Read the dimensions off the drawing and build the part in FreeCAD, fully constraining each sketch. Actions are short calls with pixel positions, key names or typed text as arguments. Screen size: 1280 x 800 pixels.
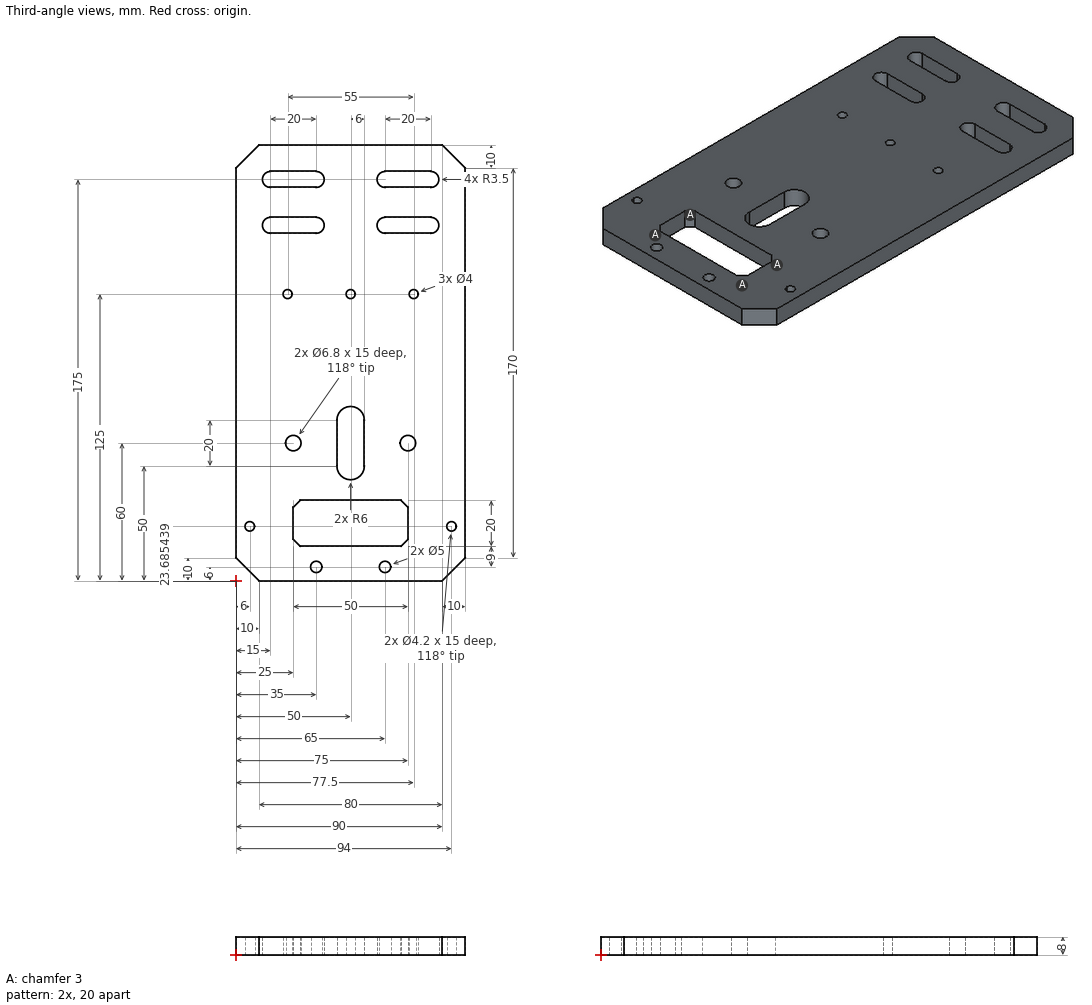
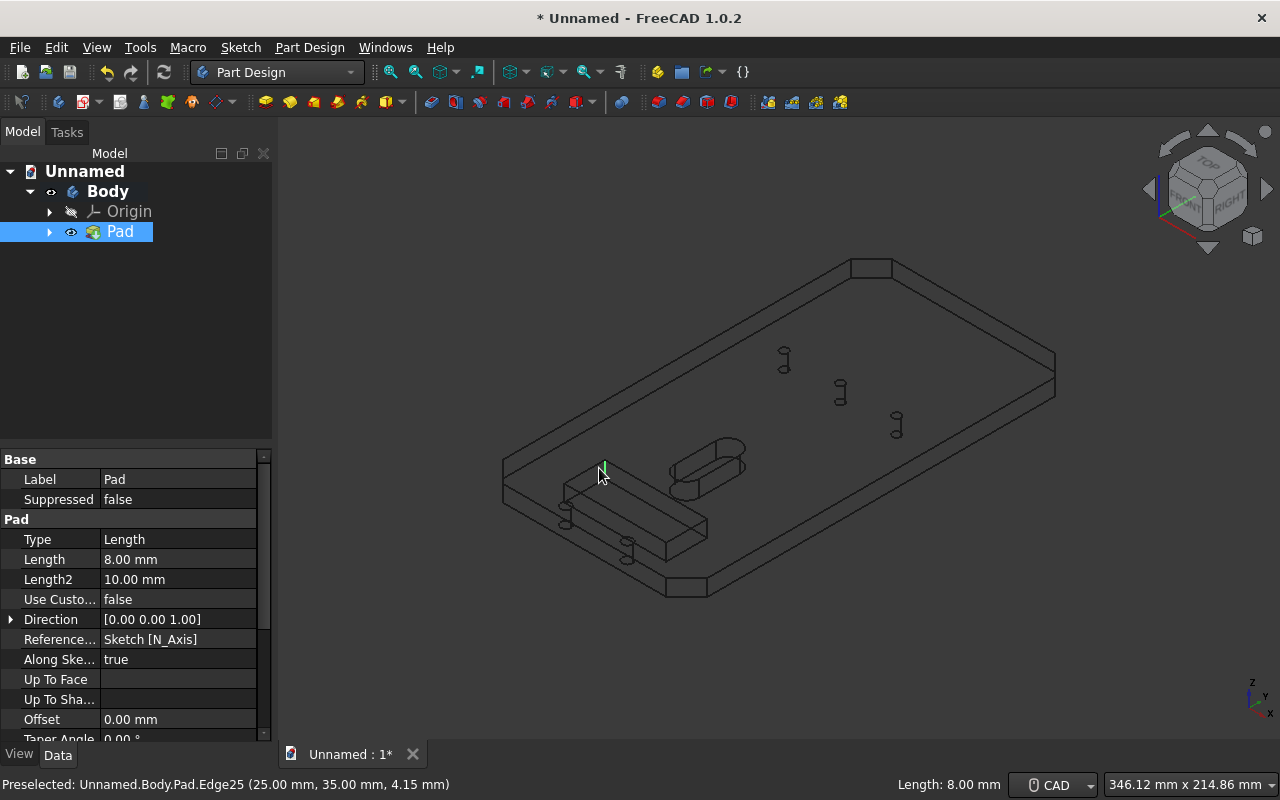
click(564, 492, ctrl)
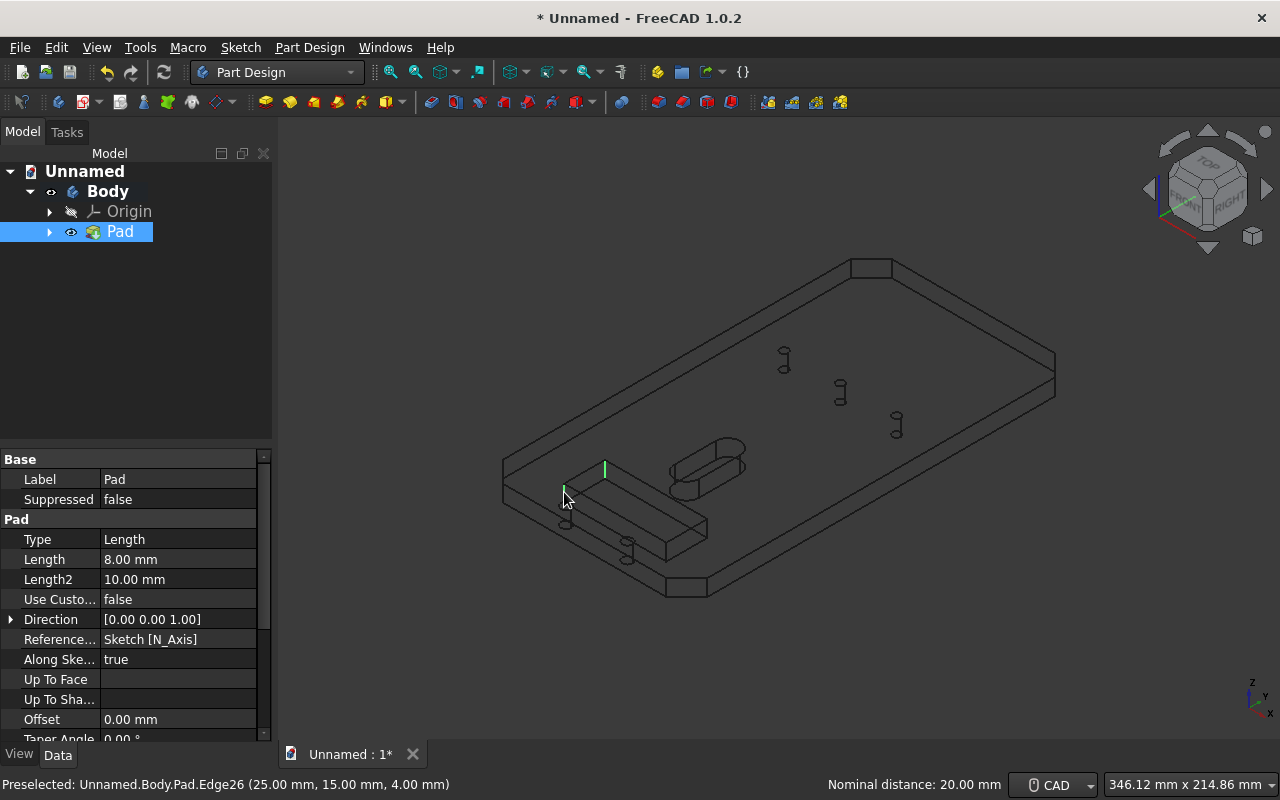
click(666, 551, ctrl)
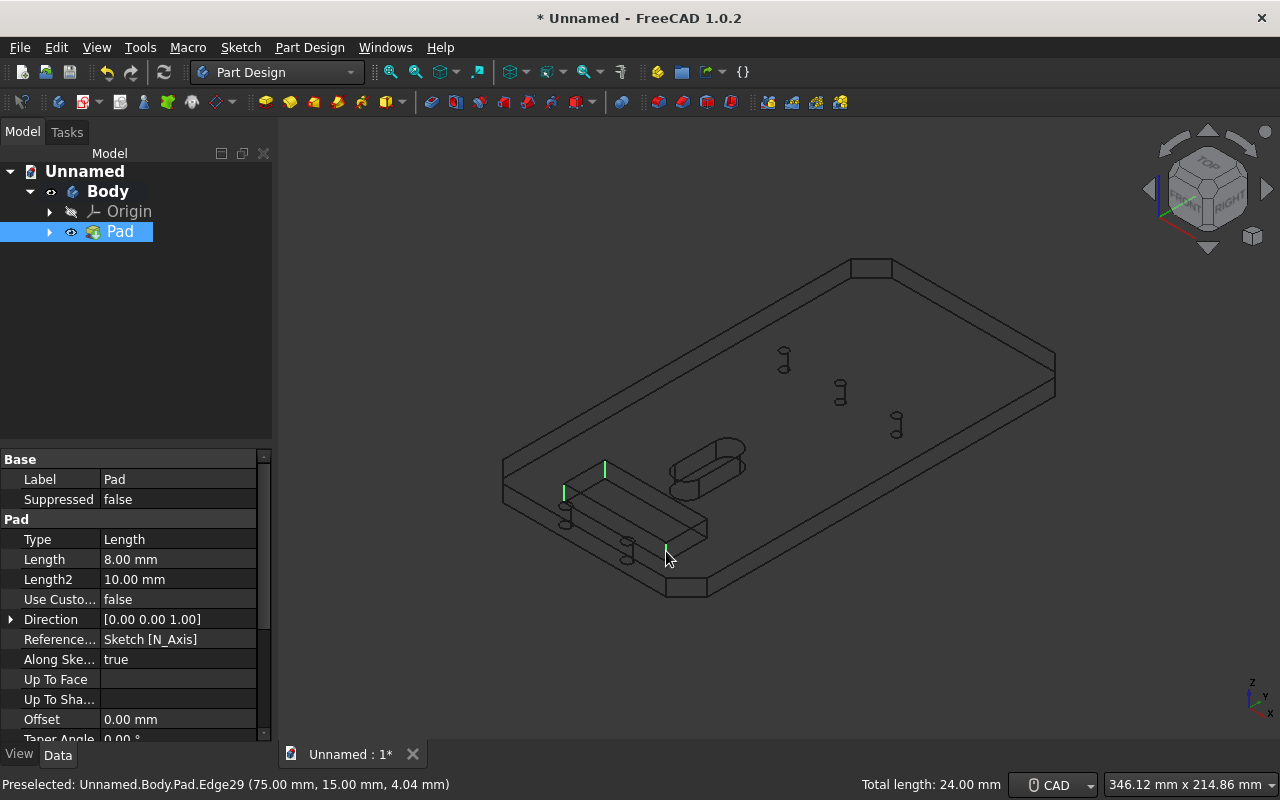
click(707, 527, ctrl)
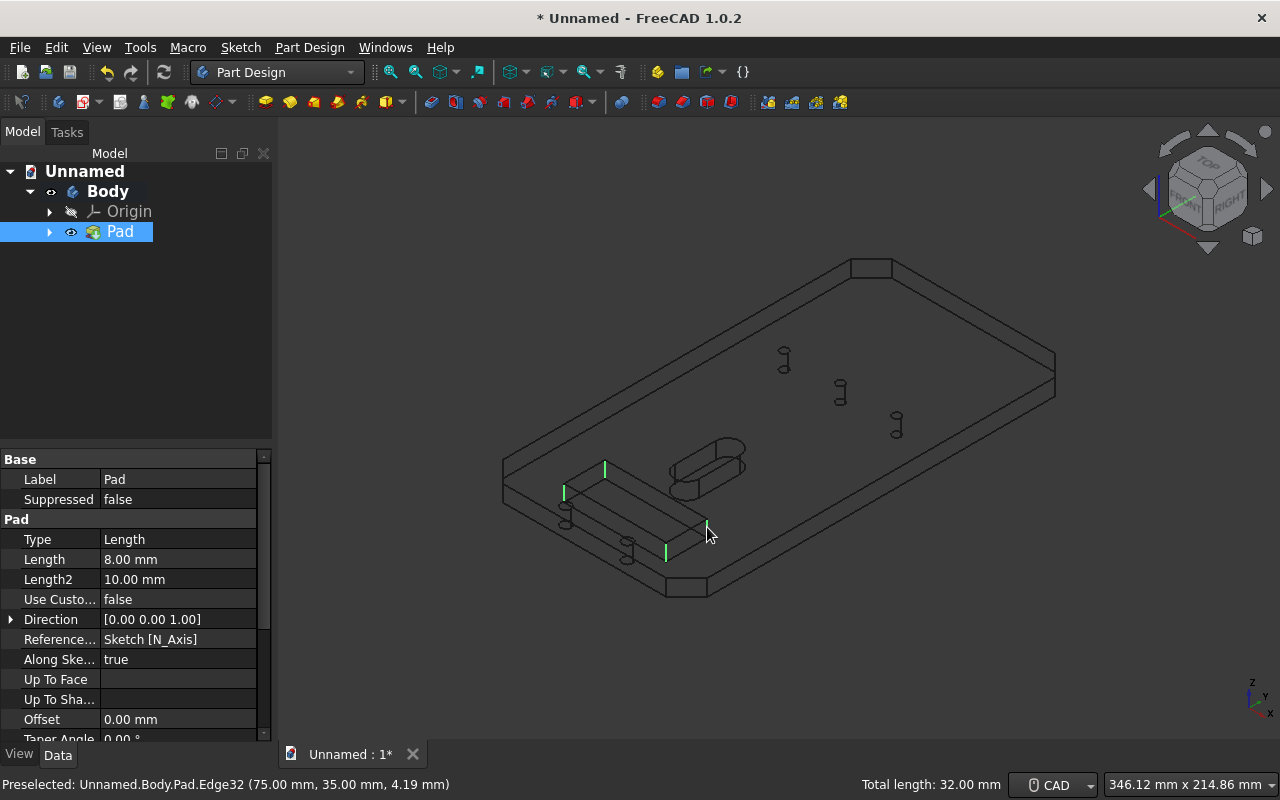
key(v)
key(1)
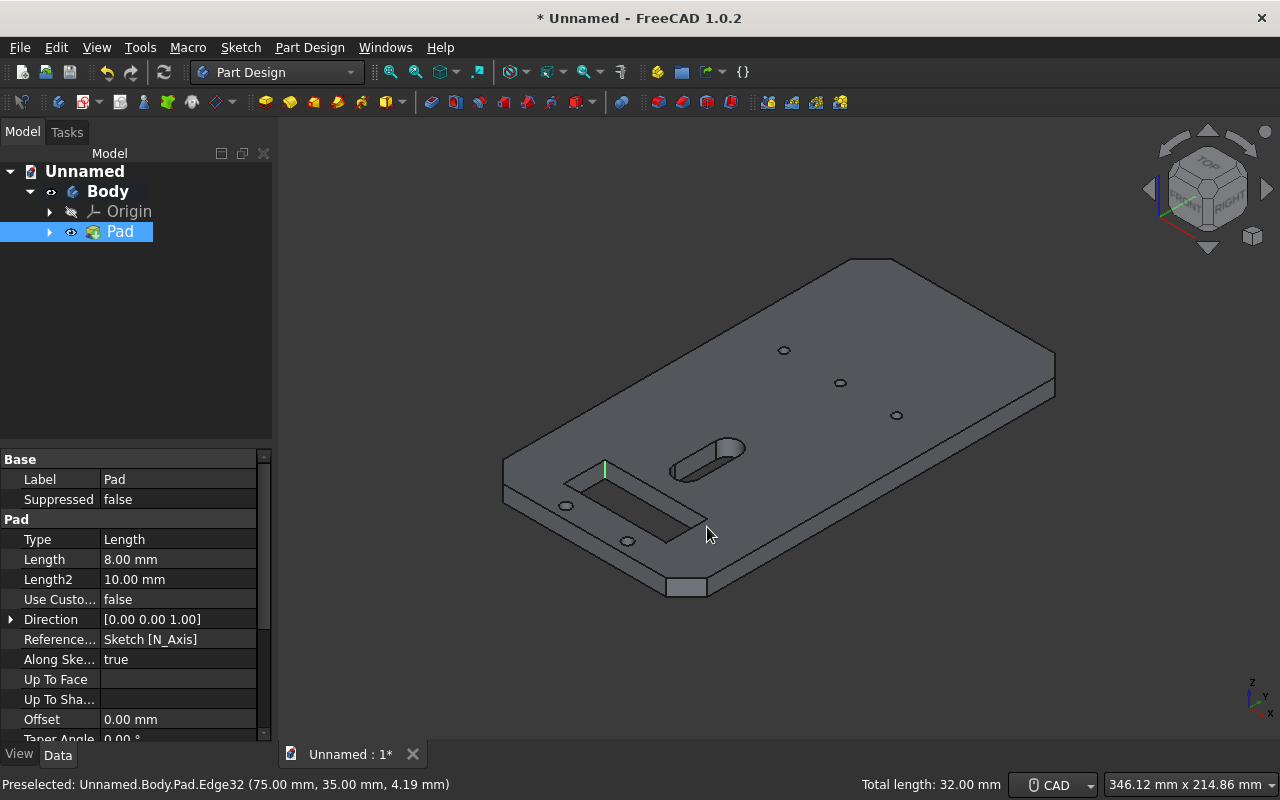
click(684, 102)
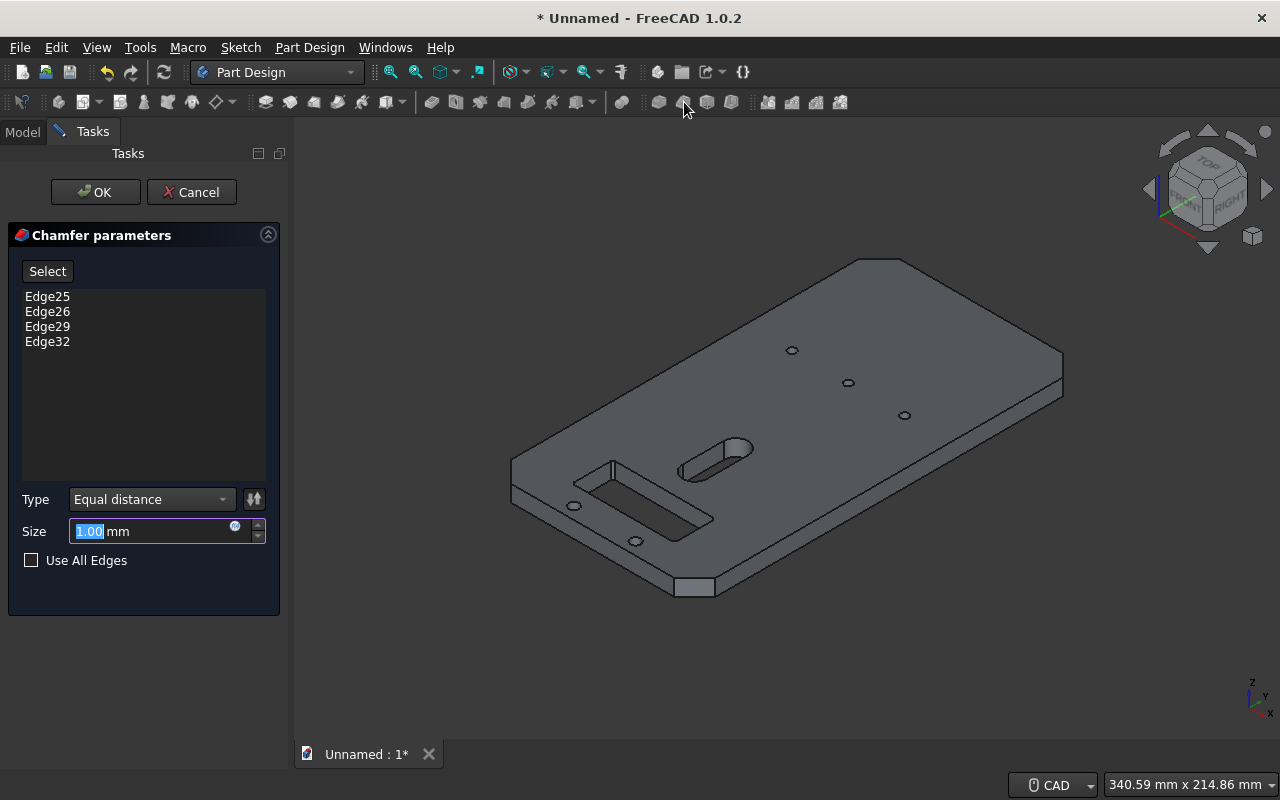
text(3)
key(Tab)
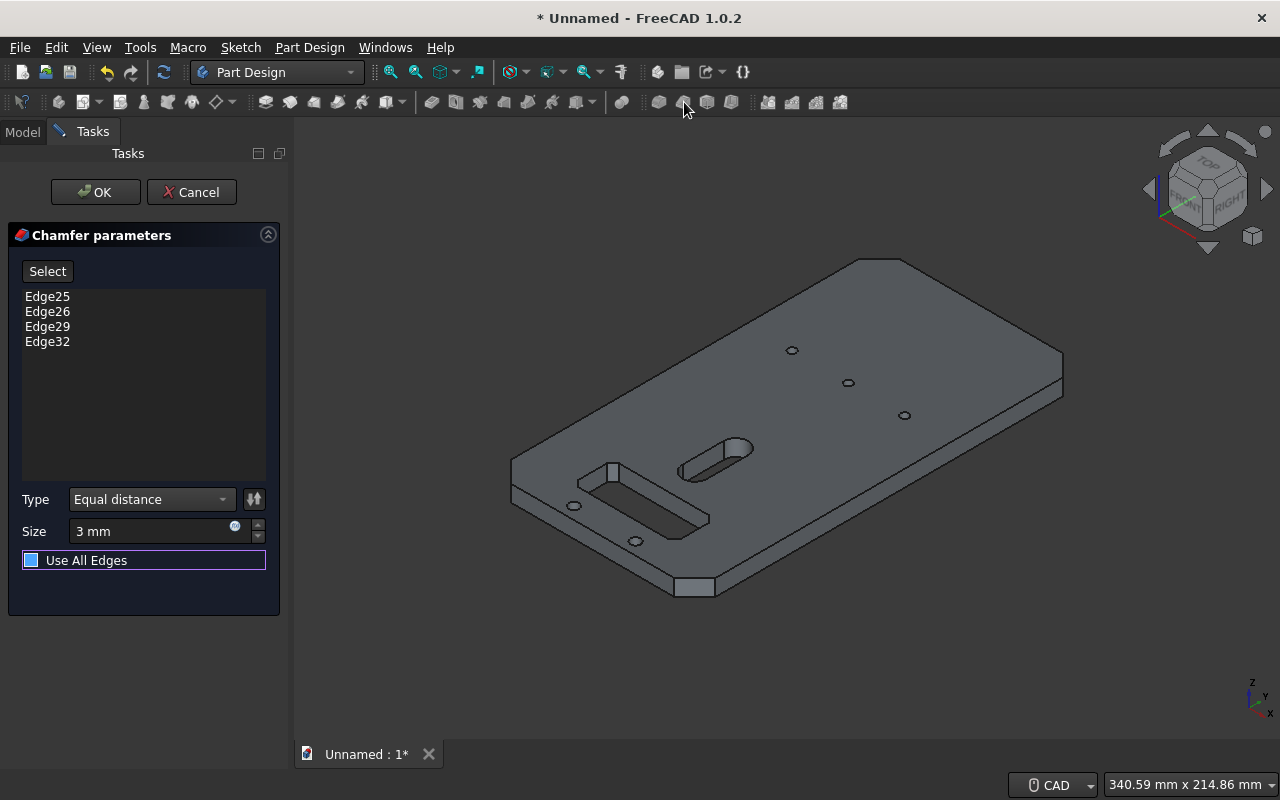
click(96, 192)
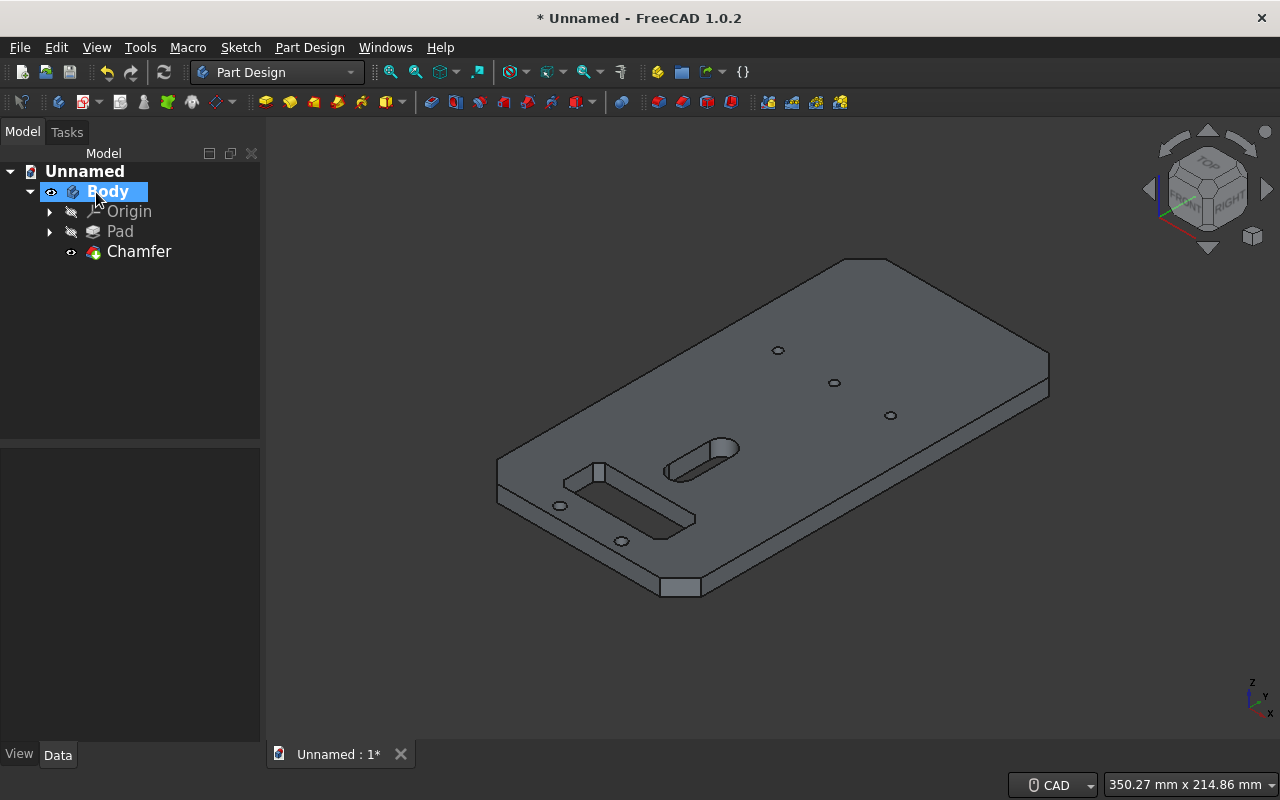
click(913, 370)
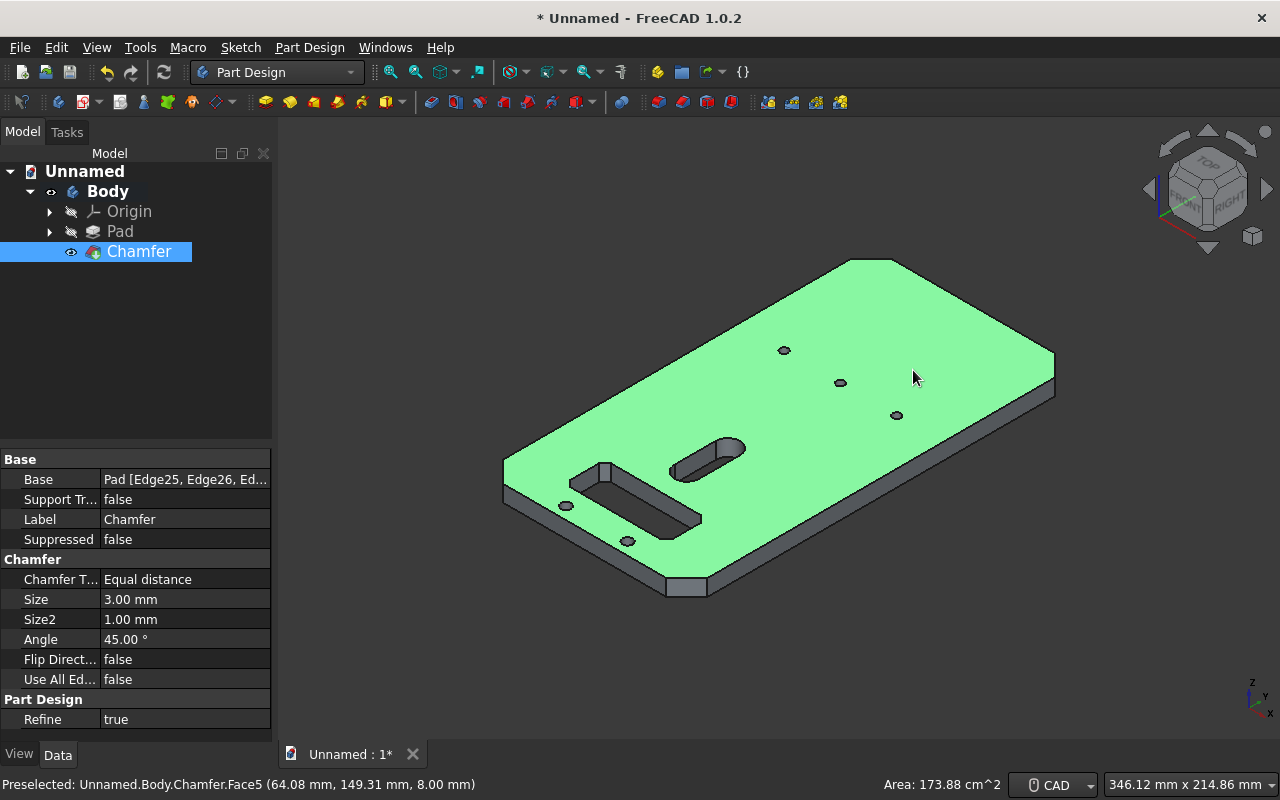
click(84, 102)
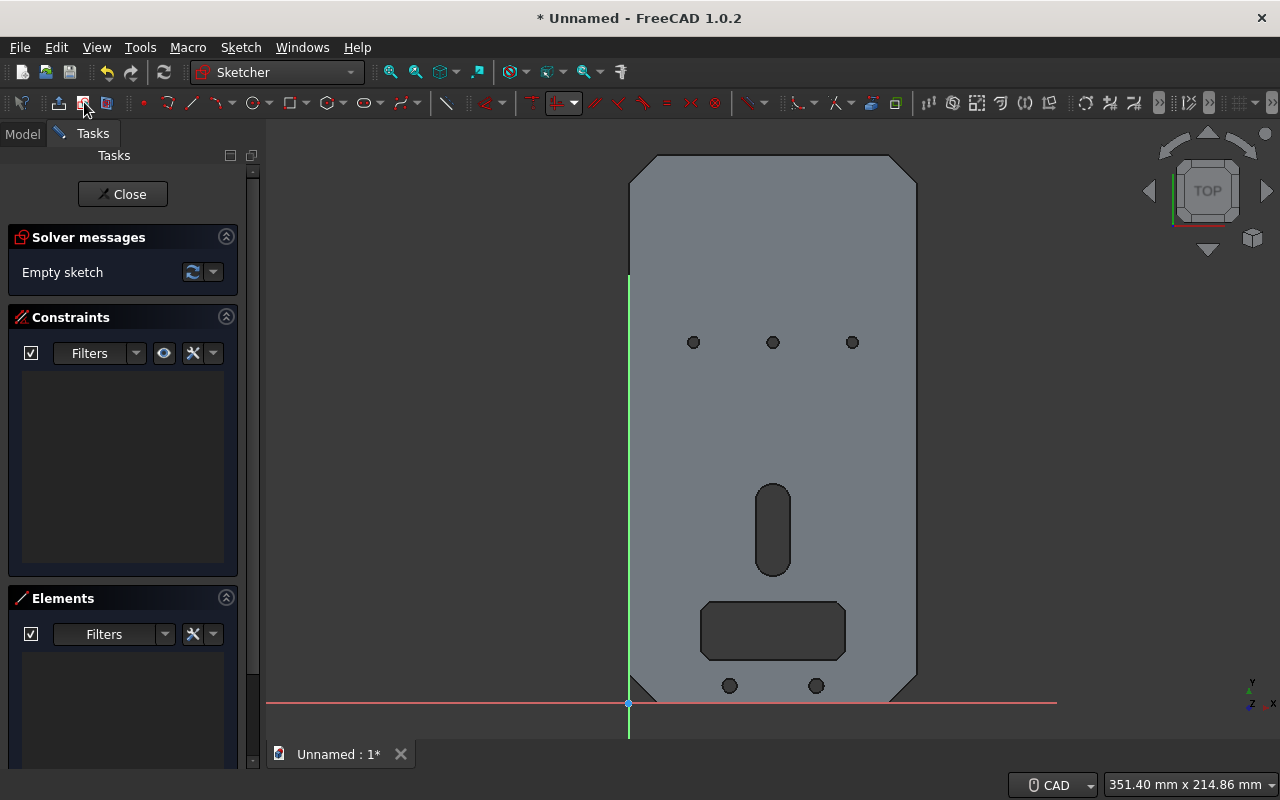
scroll(704, 429, down, 5)